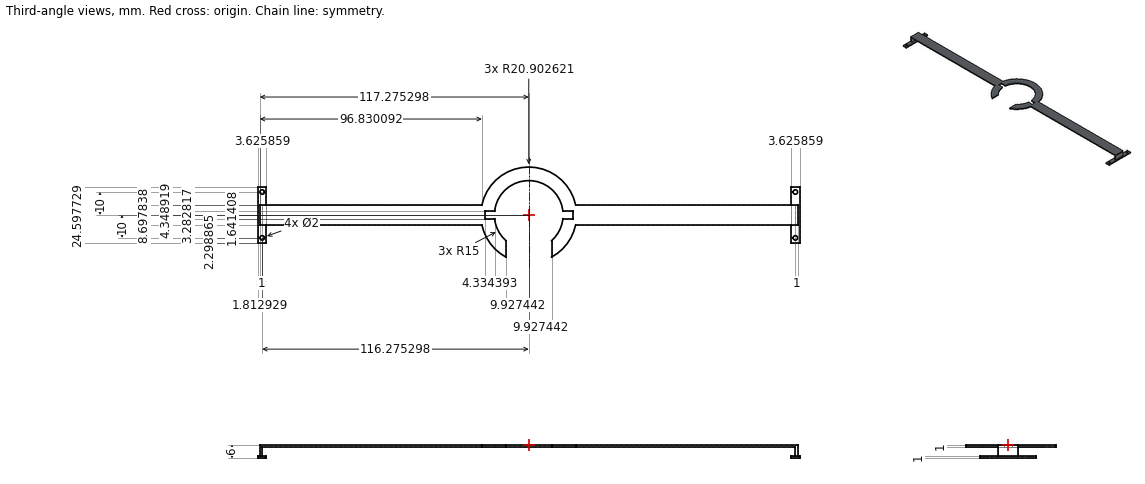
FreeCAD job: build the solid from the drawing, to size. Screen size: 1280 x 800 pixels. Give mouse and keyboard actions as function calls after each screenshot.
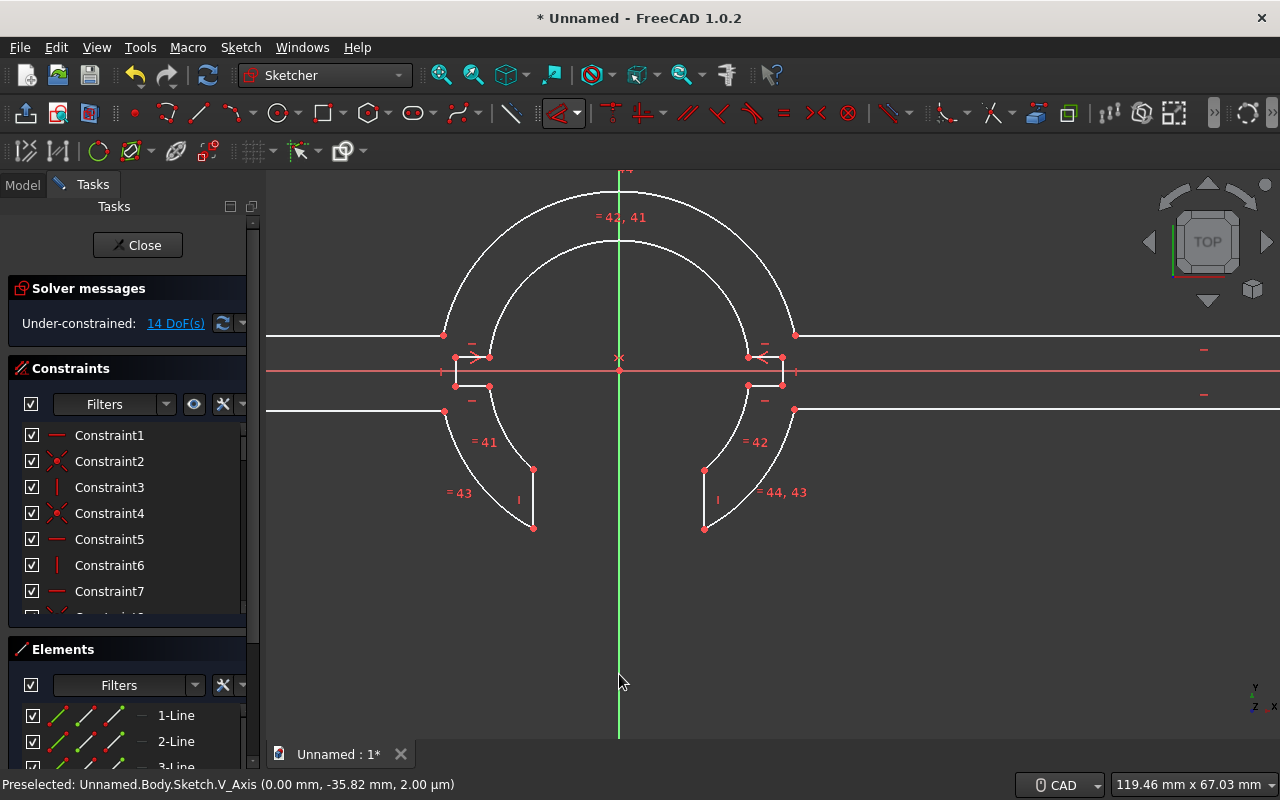
scroll(741, 495, down, 6)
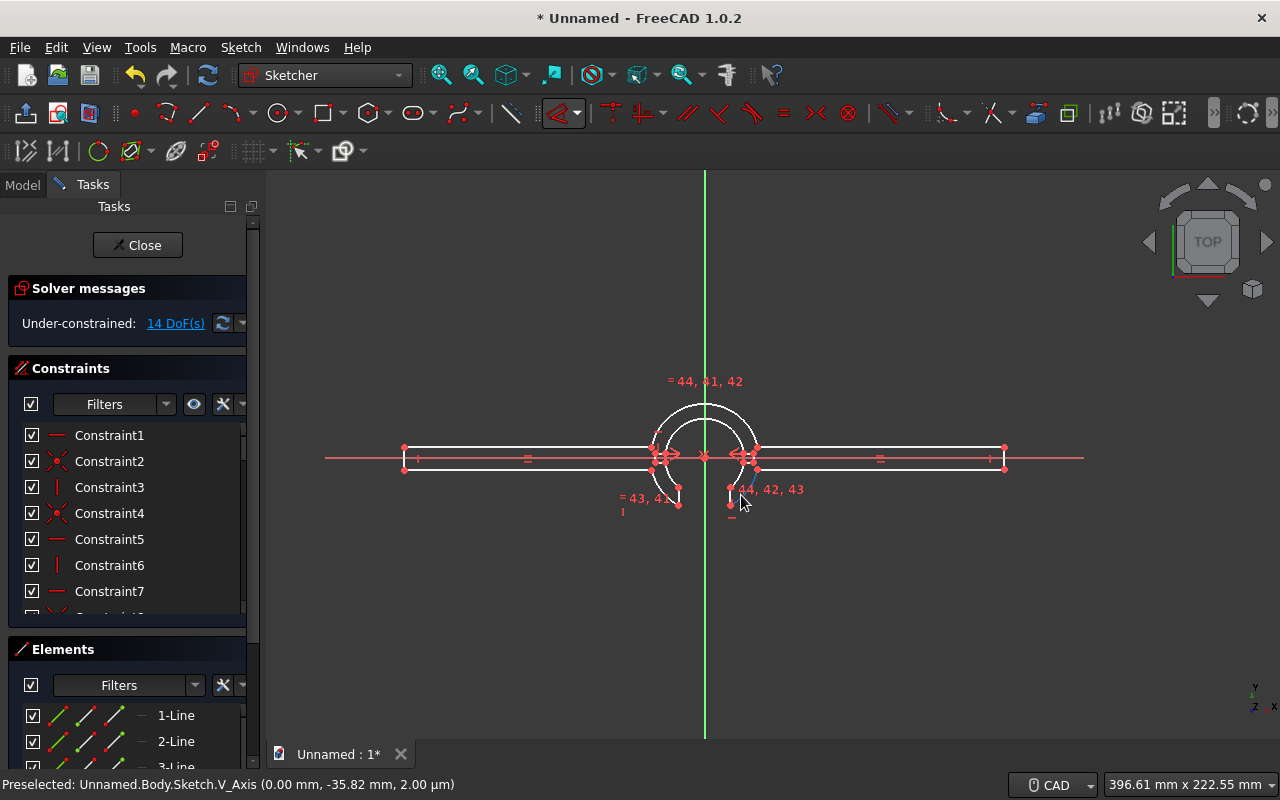
click(404, 470)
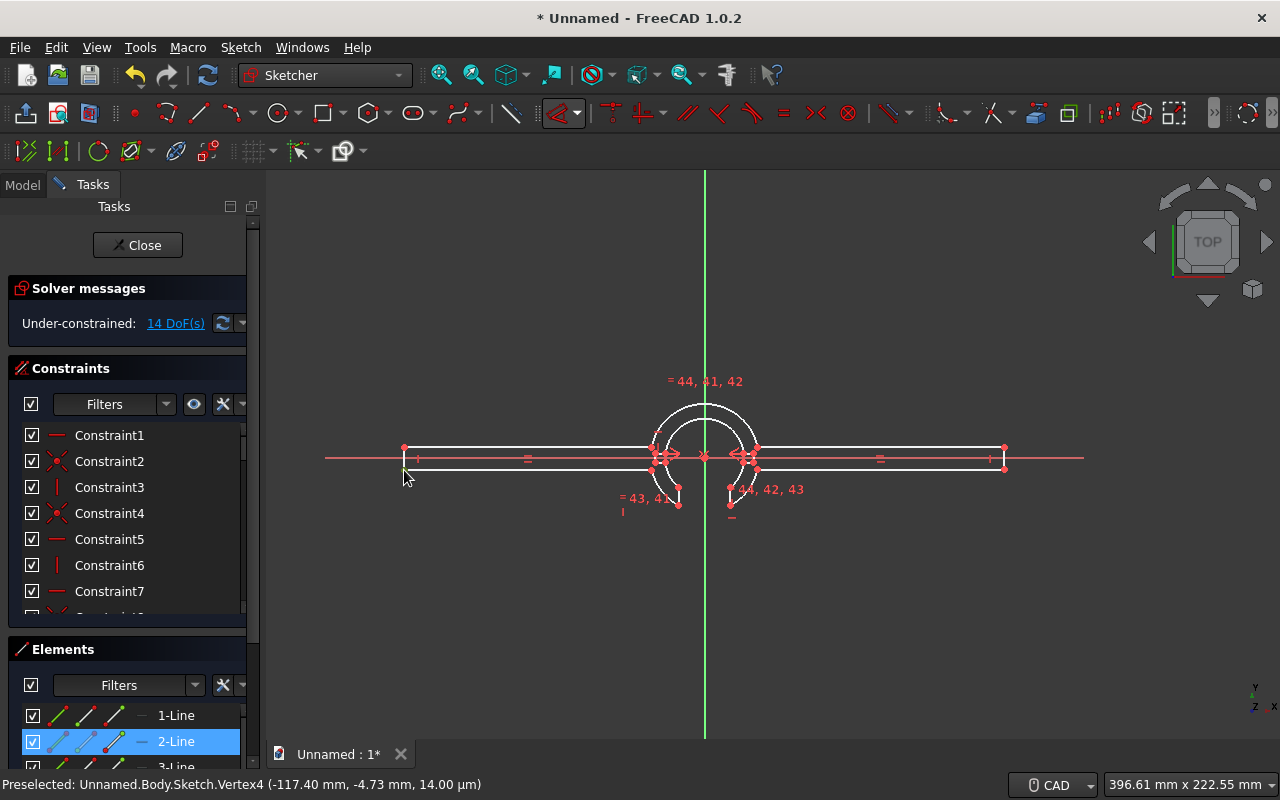
click(1004, 470)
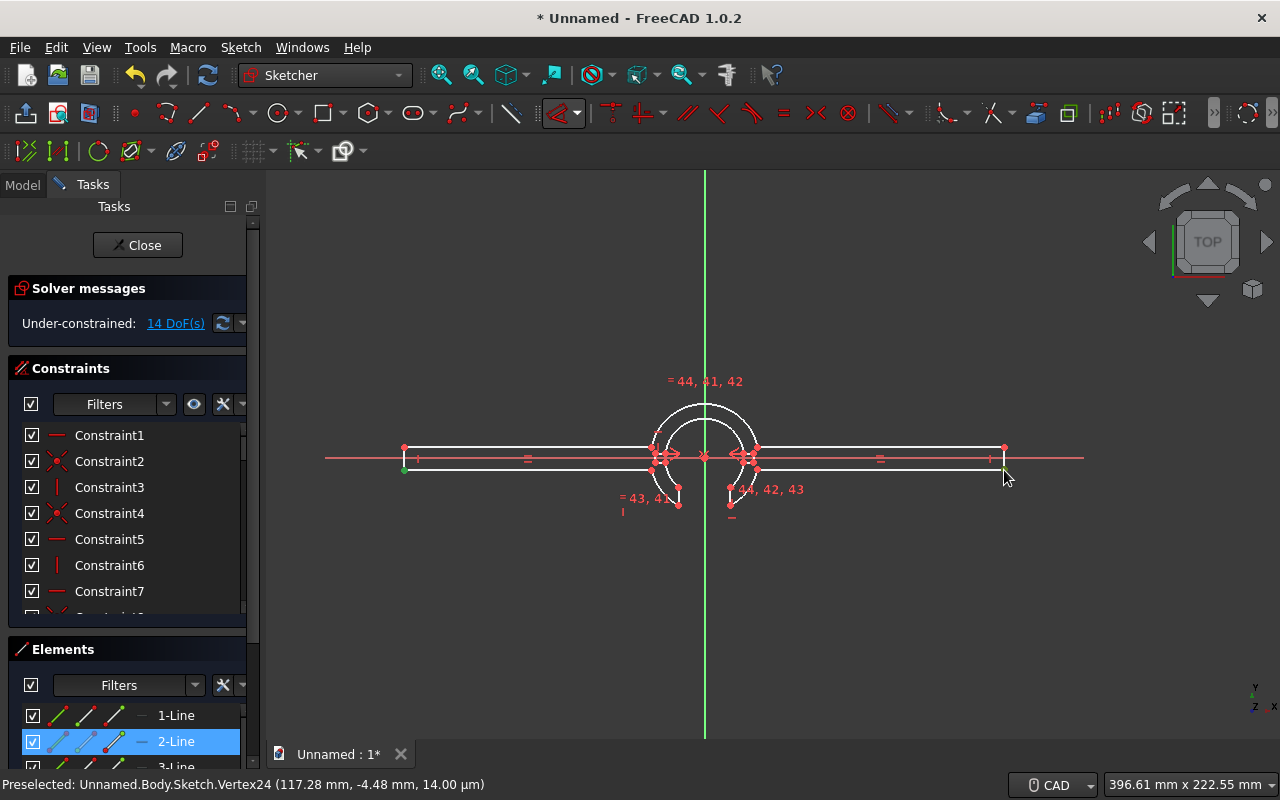
click(705, 674)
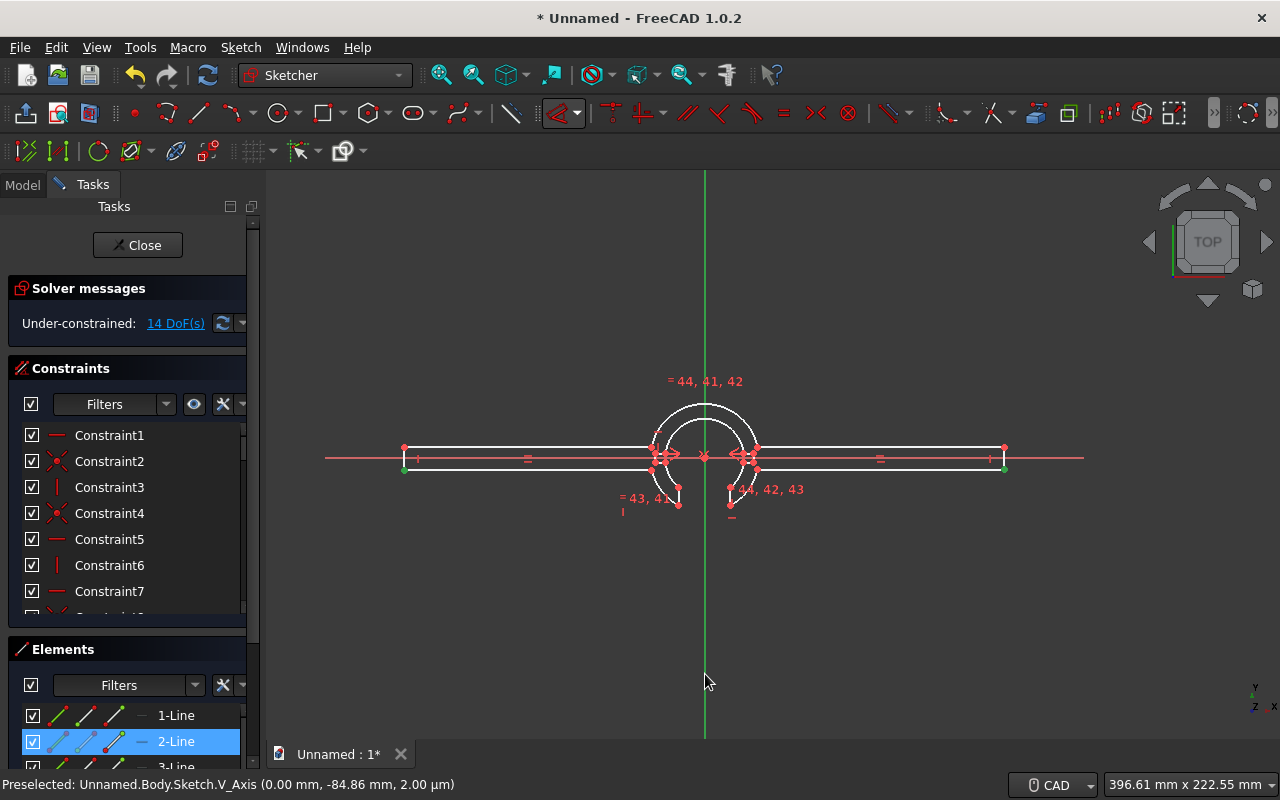
click(816, 114)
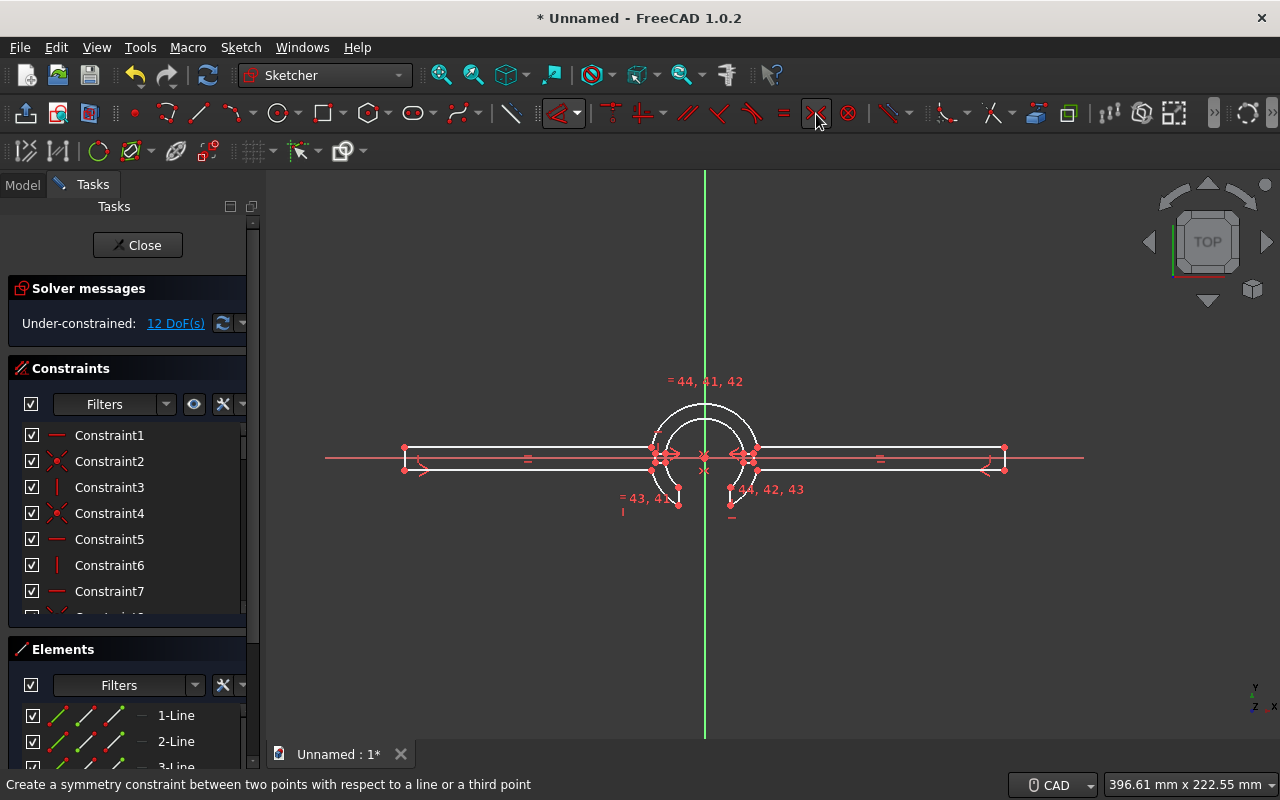
click(558, 114)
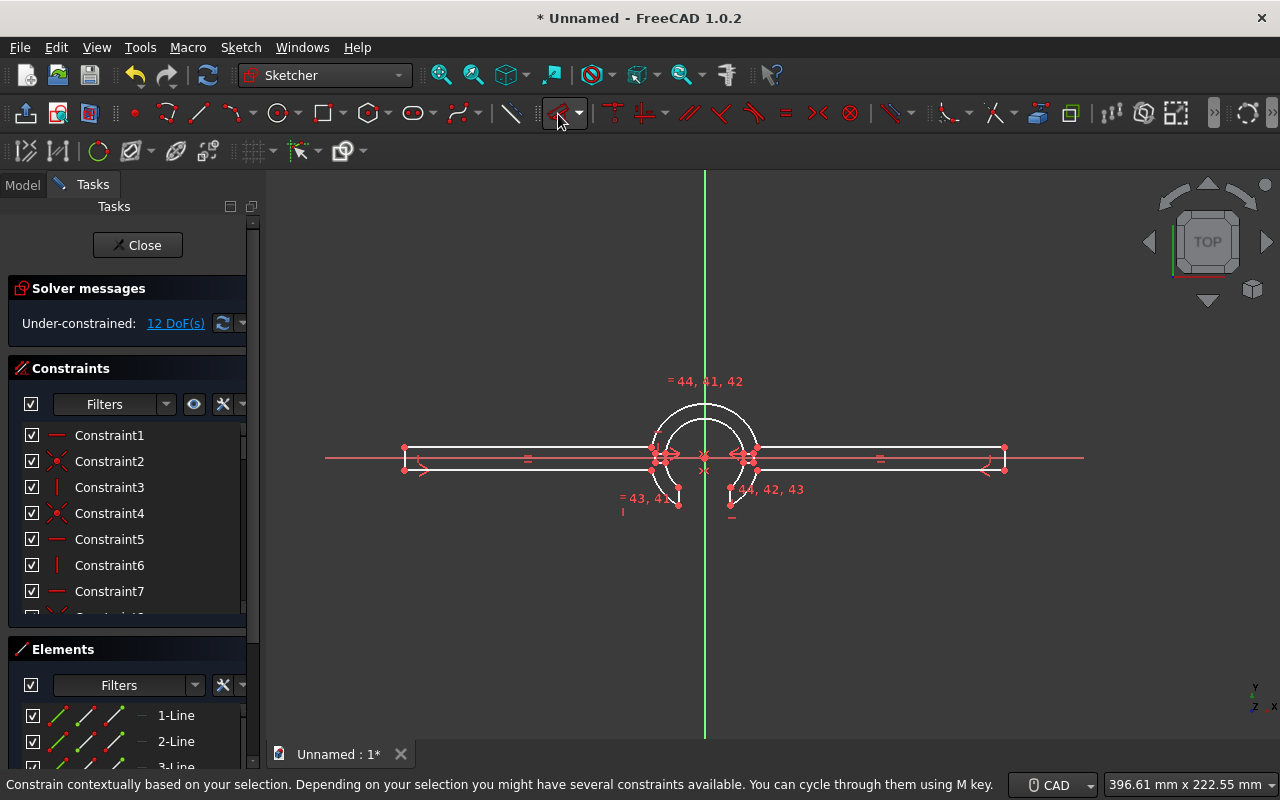
click(657, 483)
click(629, 498)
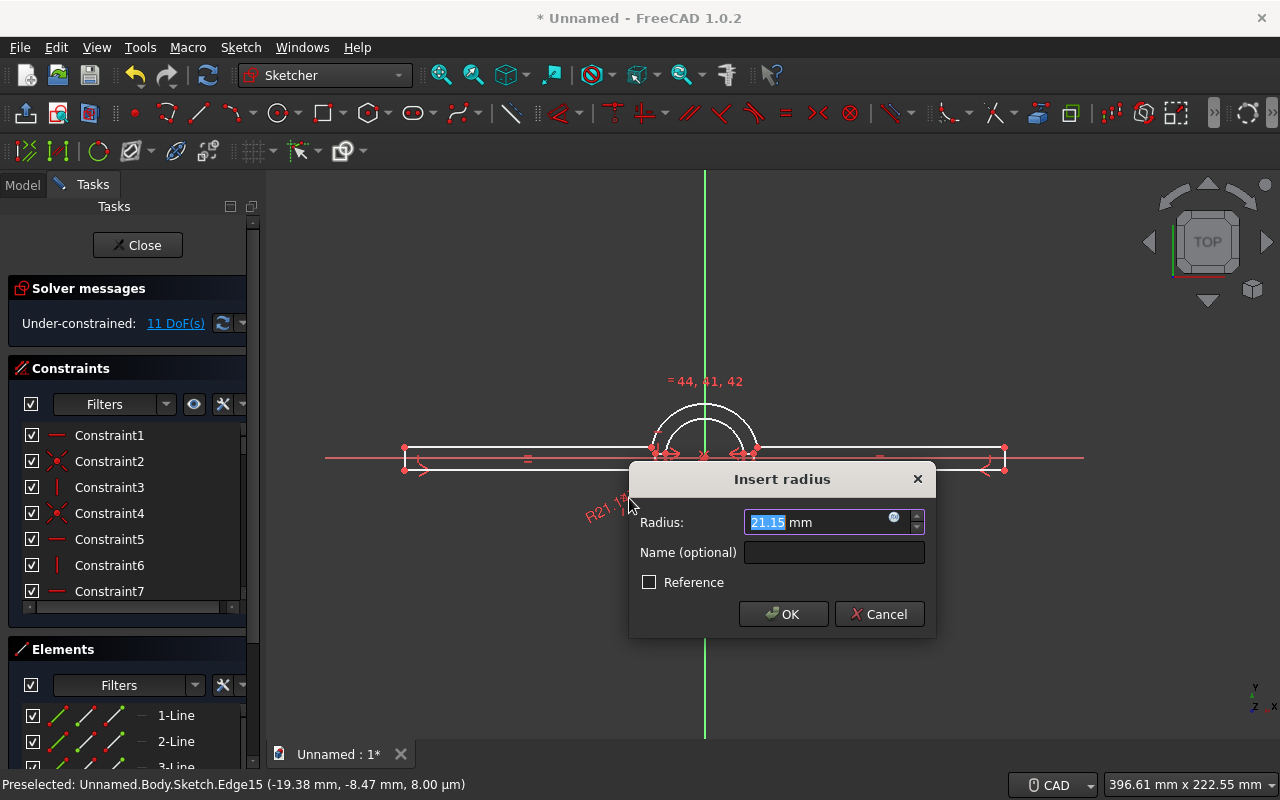
text(20.902621)
key(Return)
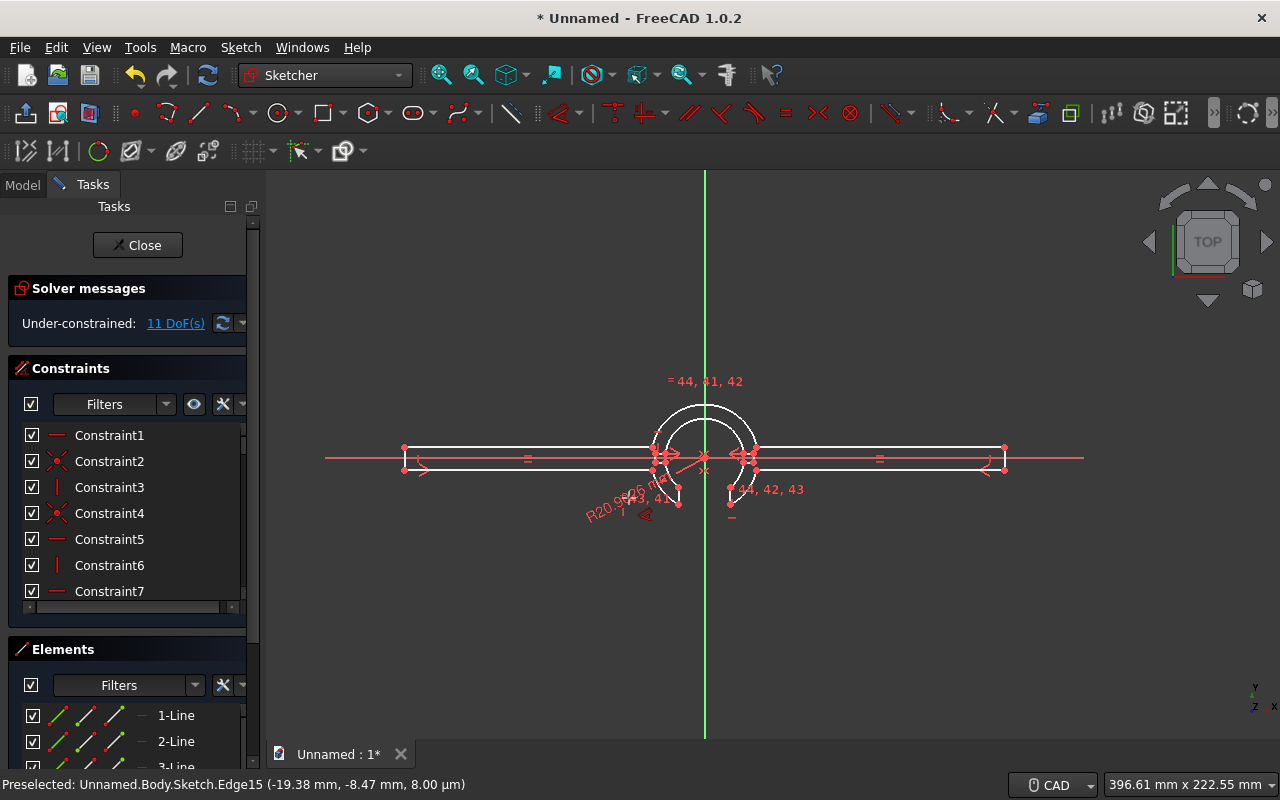
click(670, 476)
click(643, 423)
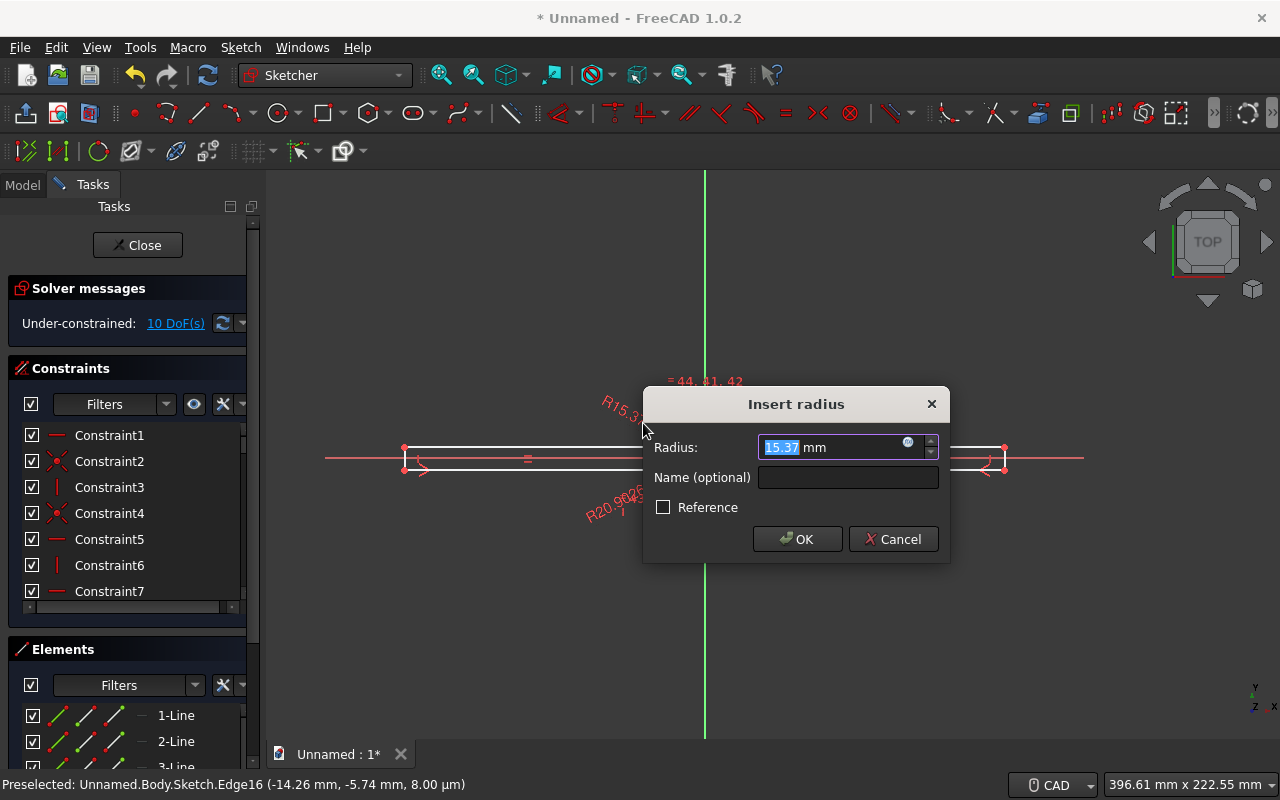
text(15)
key(Return)